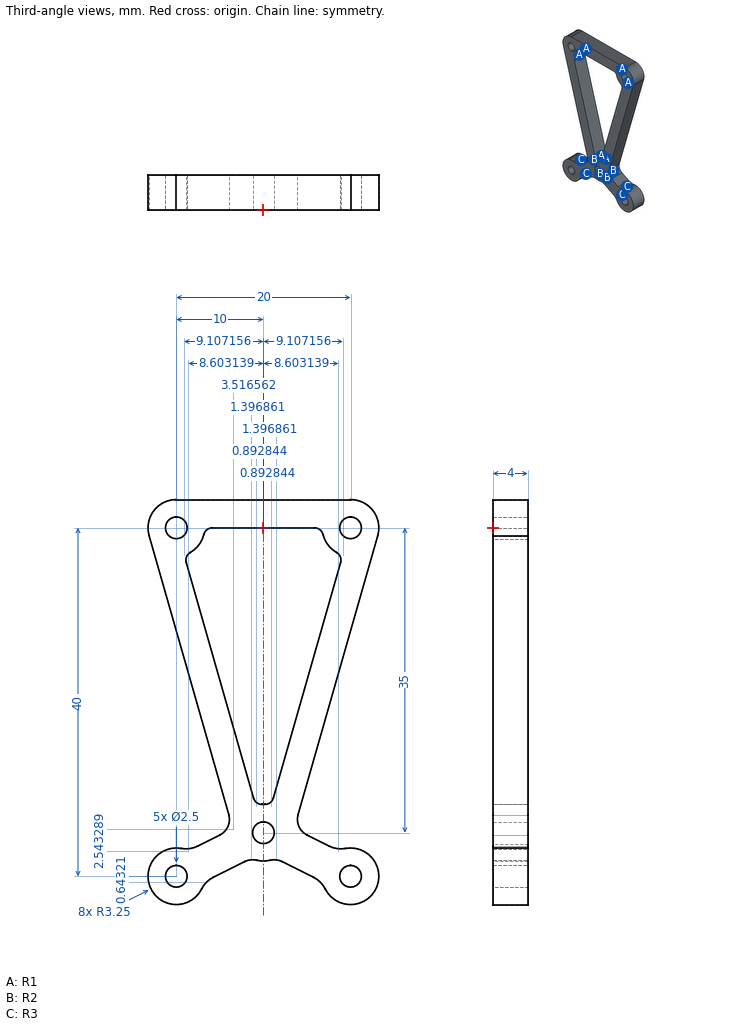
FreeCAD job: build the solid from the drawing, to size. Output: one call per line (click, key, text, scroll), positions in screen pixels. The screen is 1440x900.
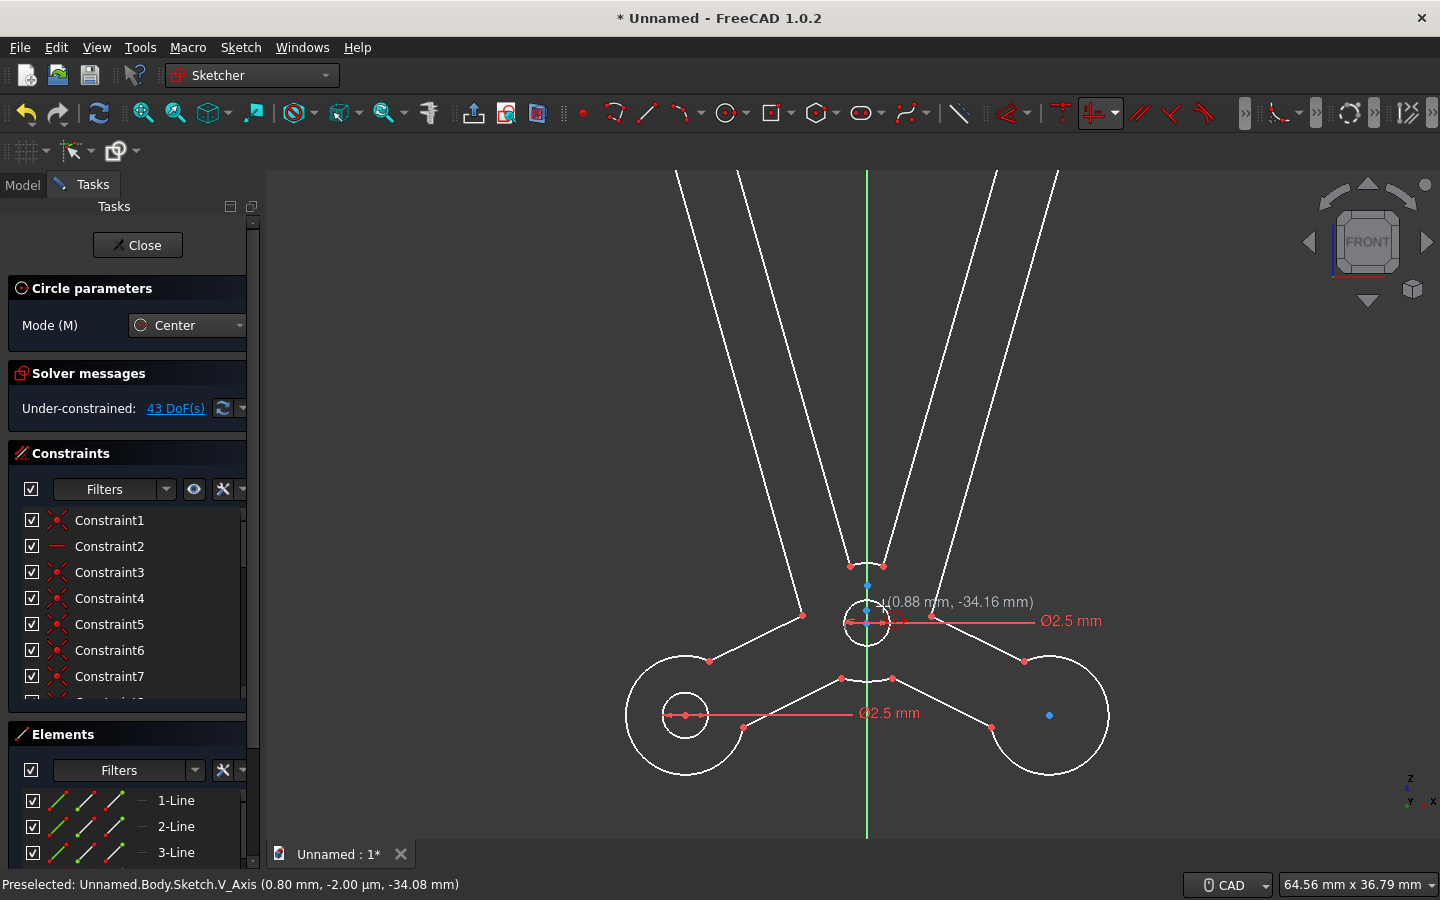
scroll(684, 713, down, 3)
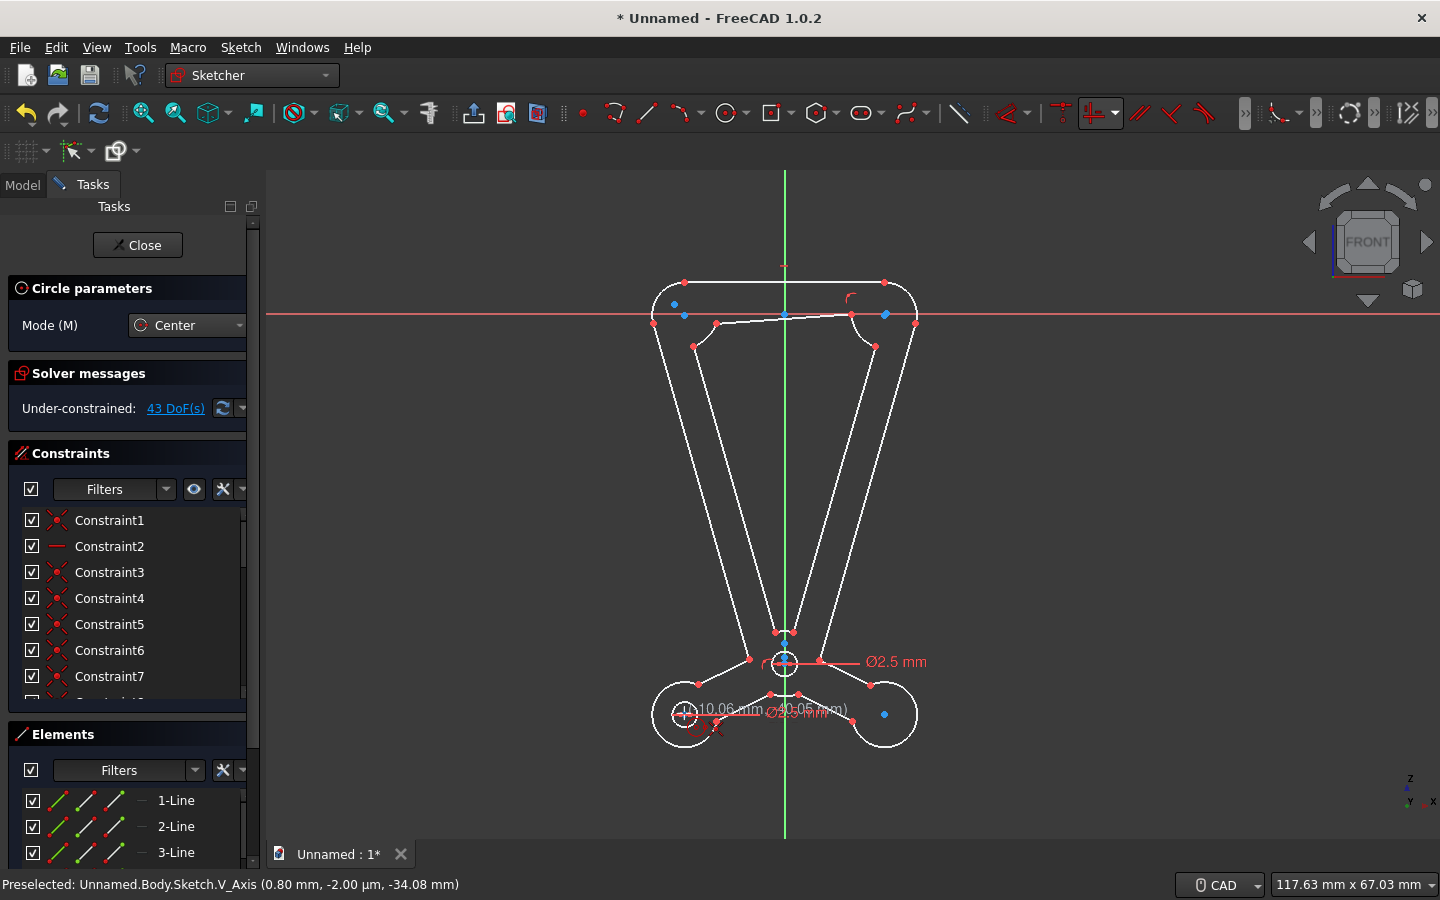
scroll(685, 314, up, 3)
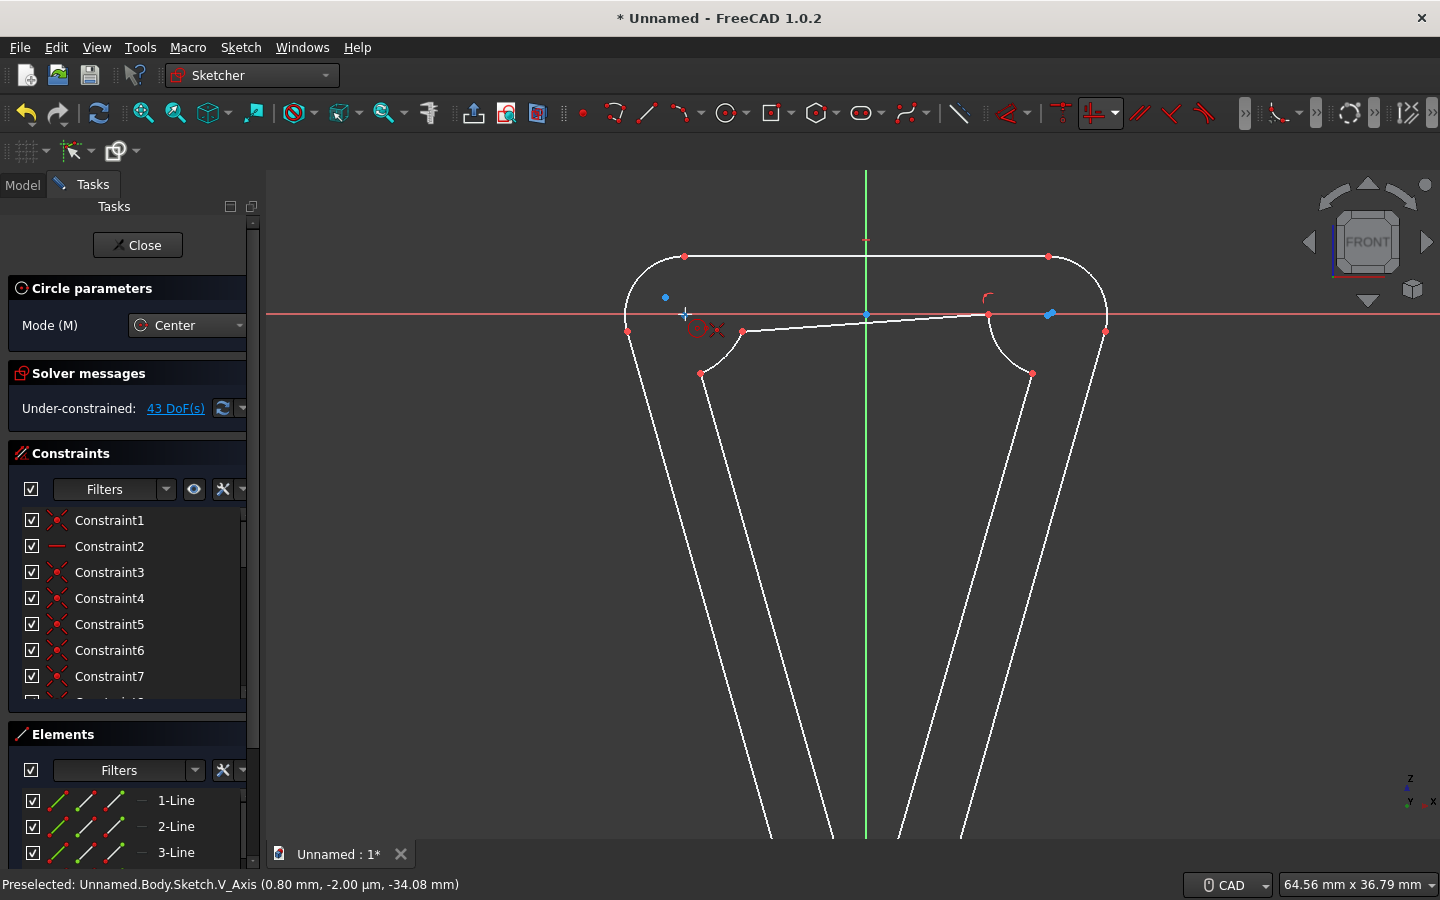
click(684, 314)
move(700, 298)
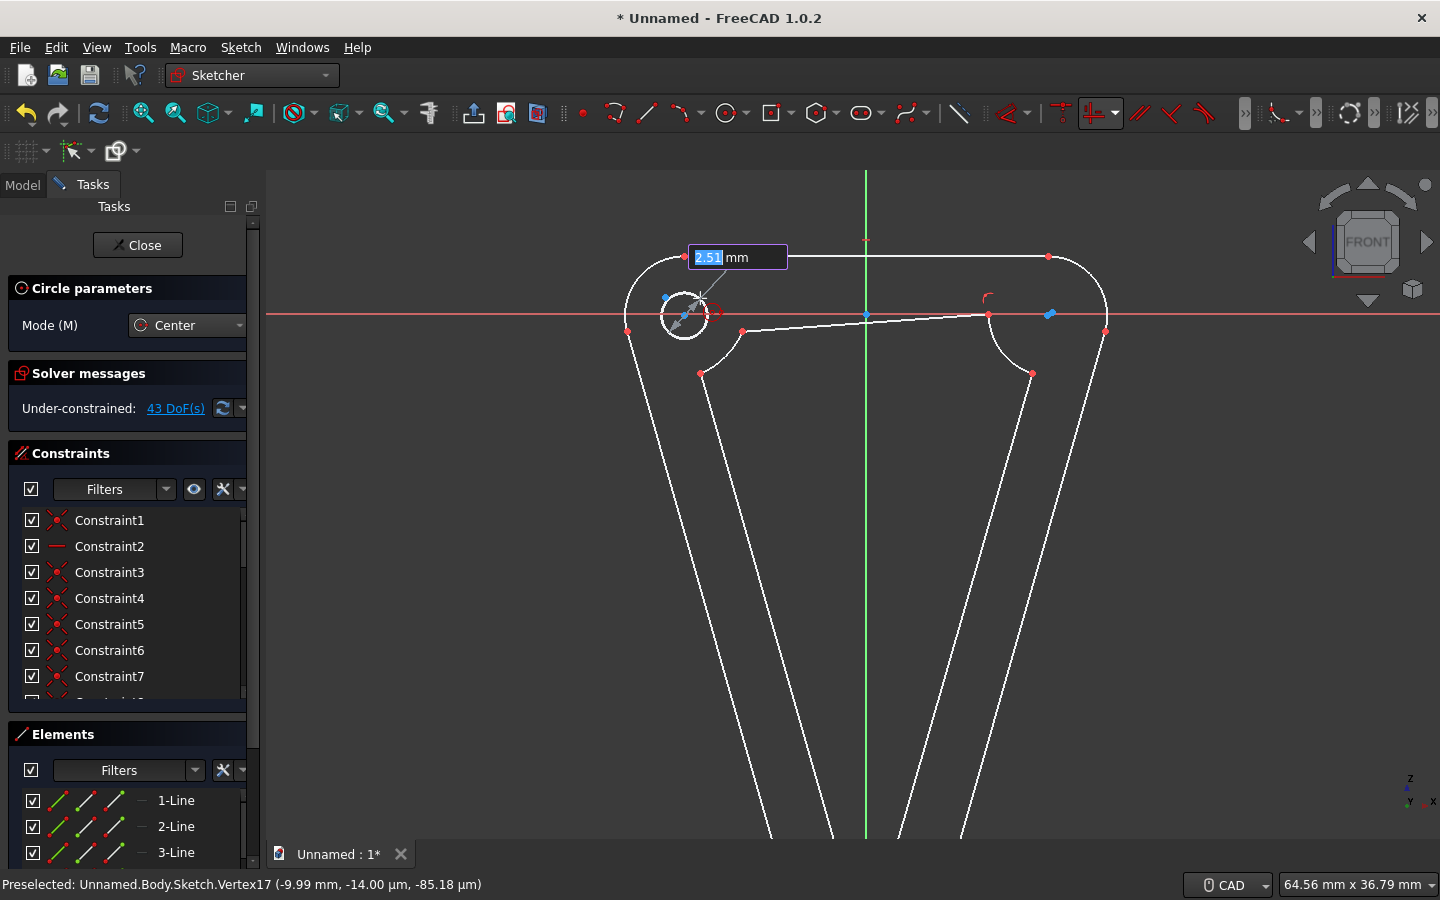
text(2.5)
key(Return)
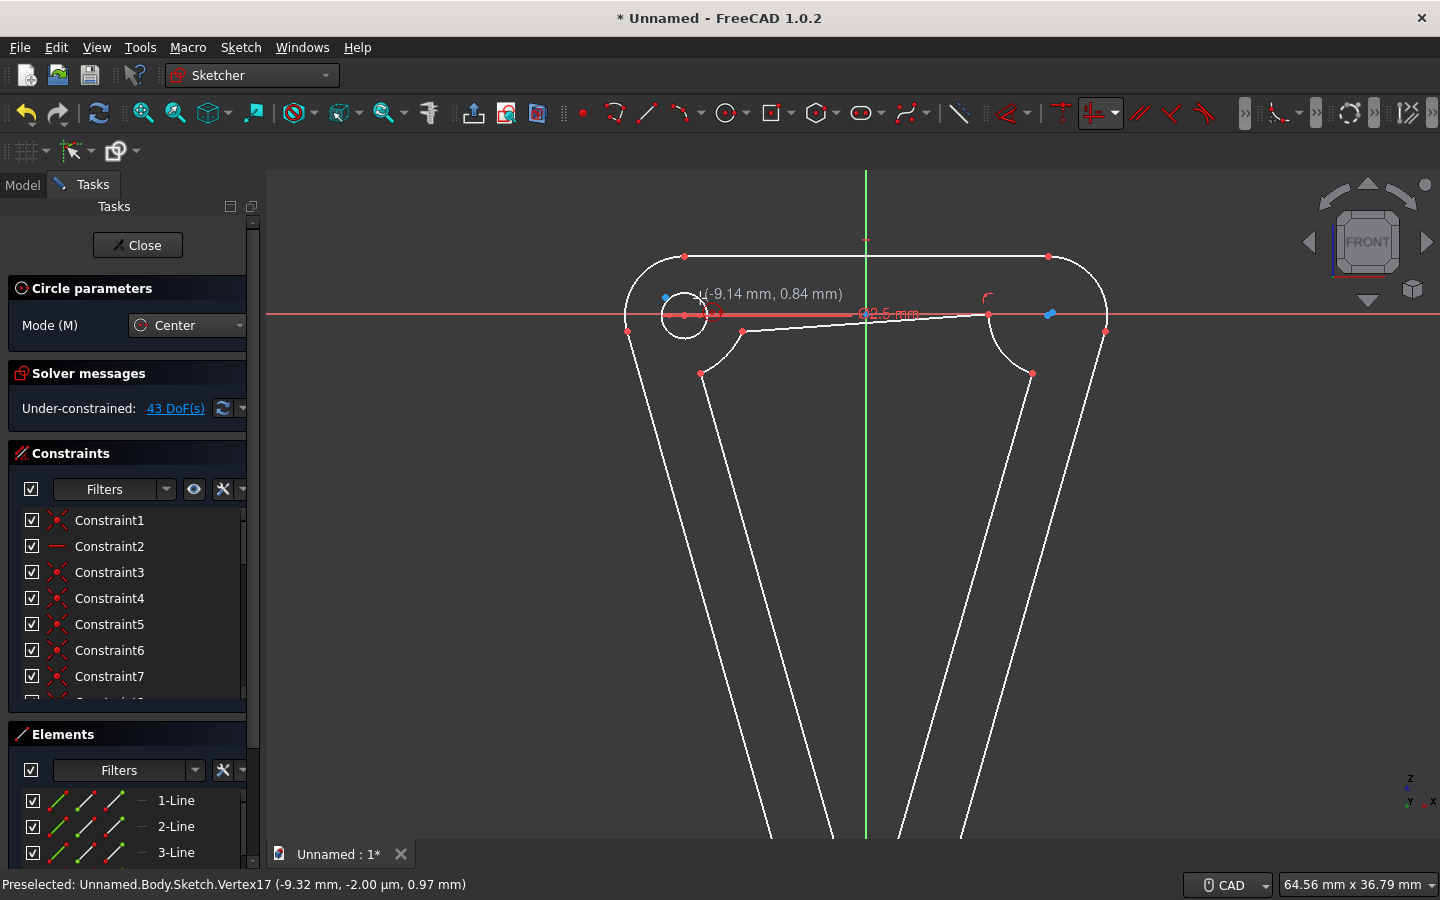
scroll(685, 313, down, 3)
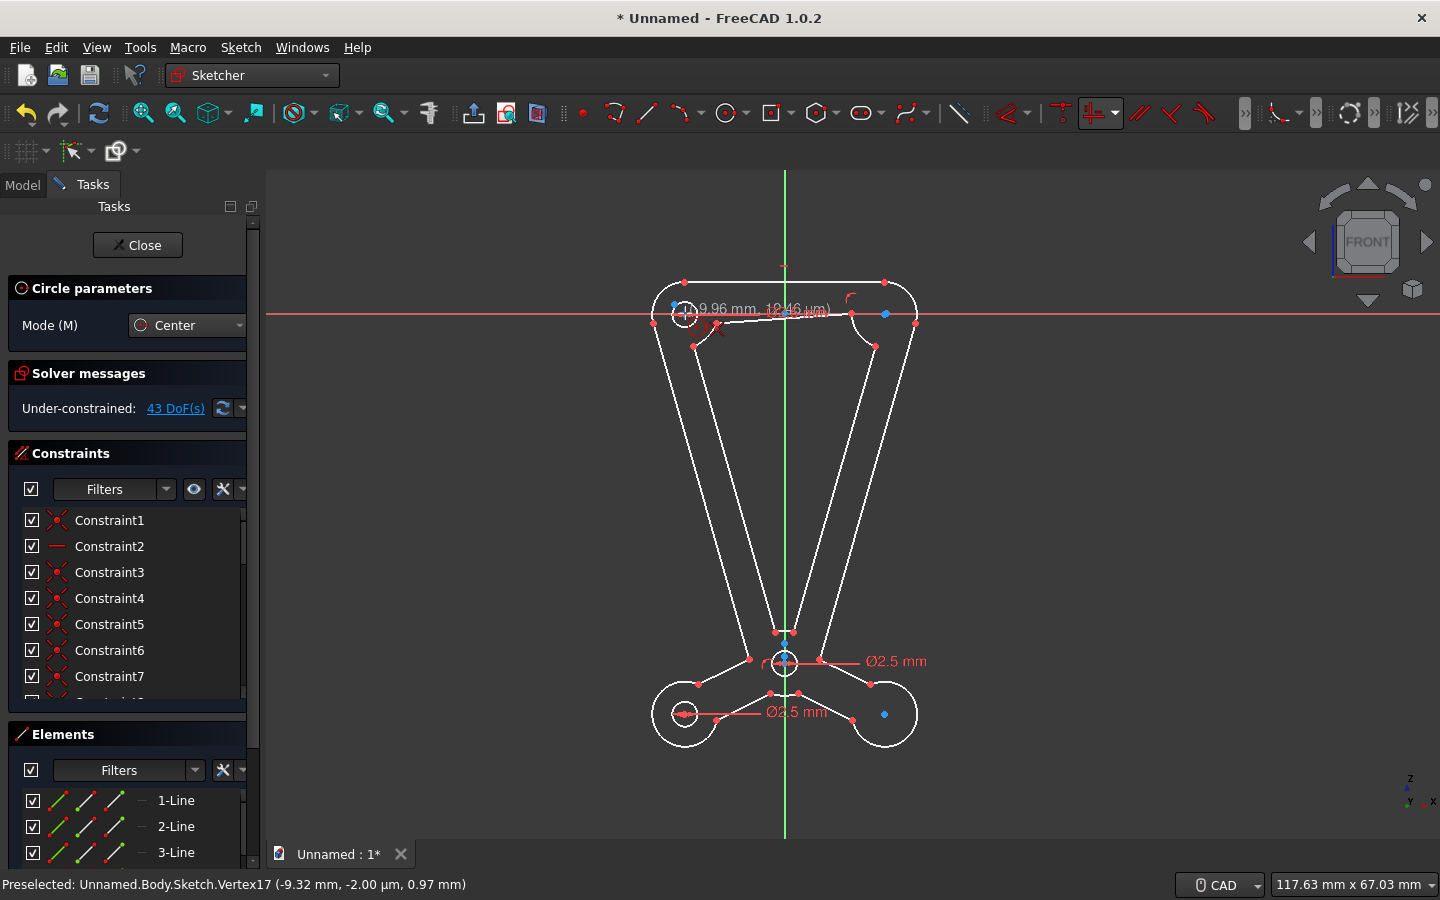
scroll(884, 713, up, 3)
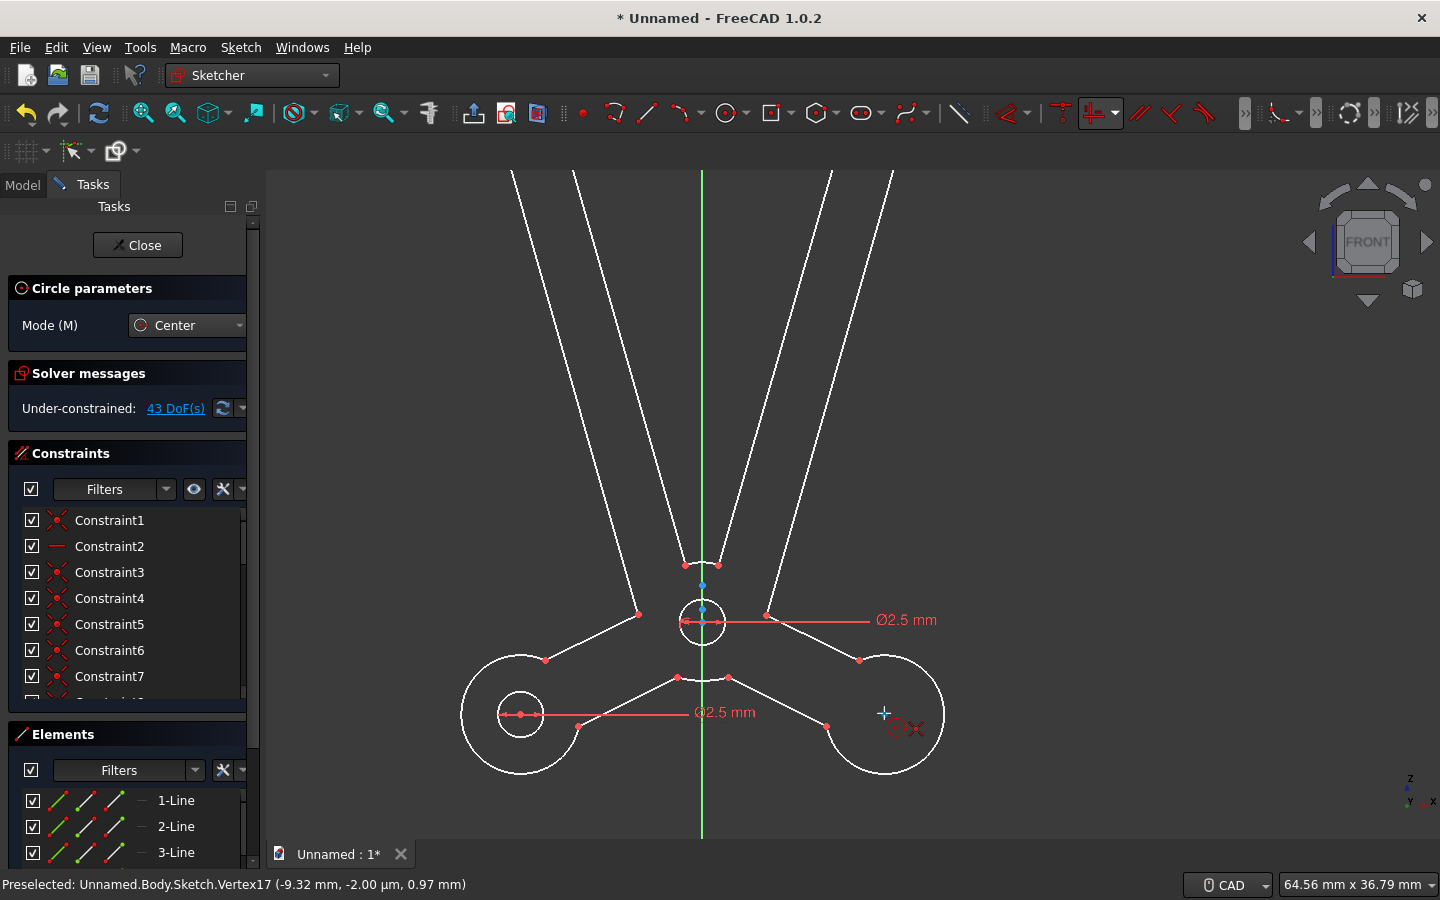
click(884, 712)
move(900, 696)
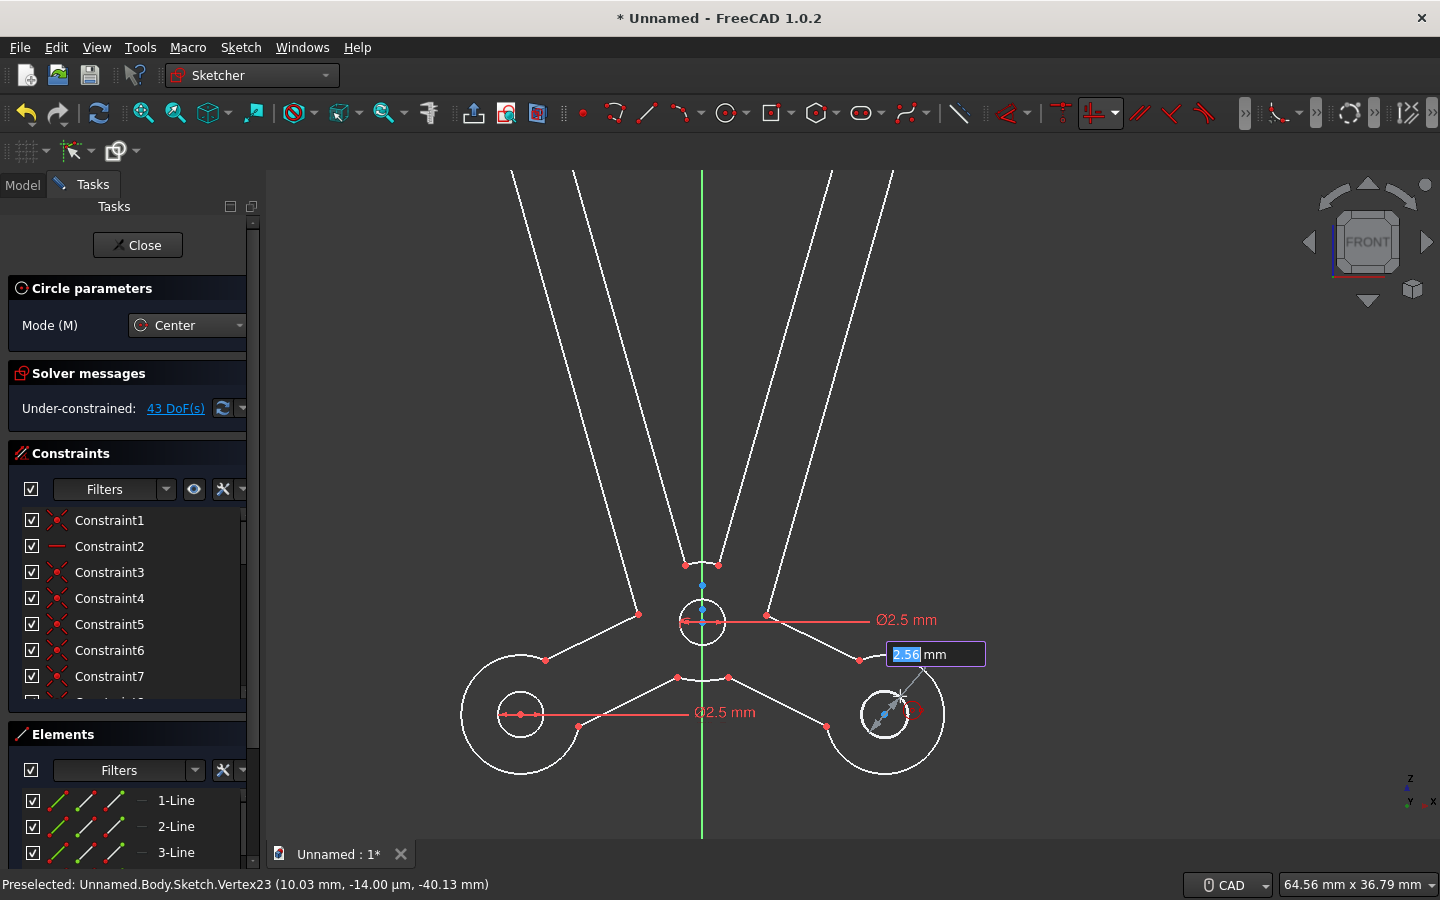
text(2.5)
key(Return)